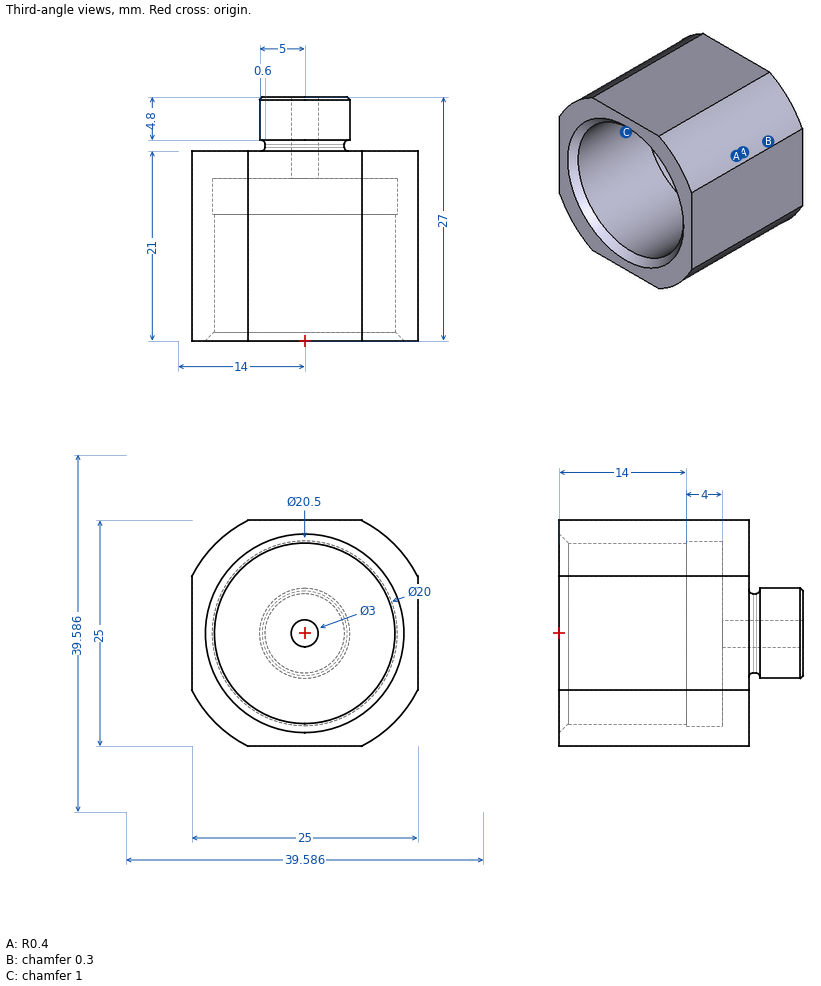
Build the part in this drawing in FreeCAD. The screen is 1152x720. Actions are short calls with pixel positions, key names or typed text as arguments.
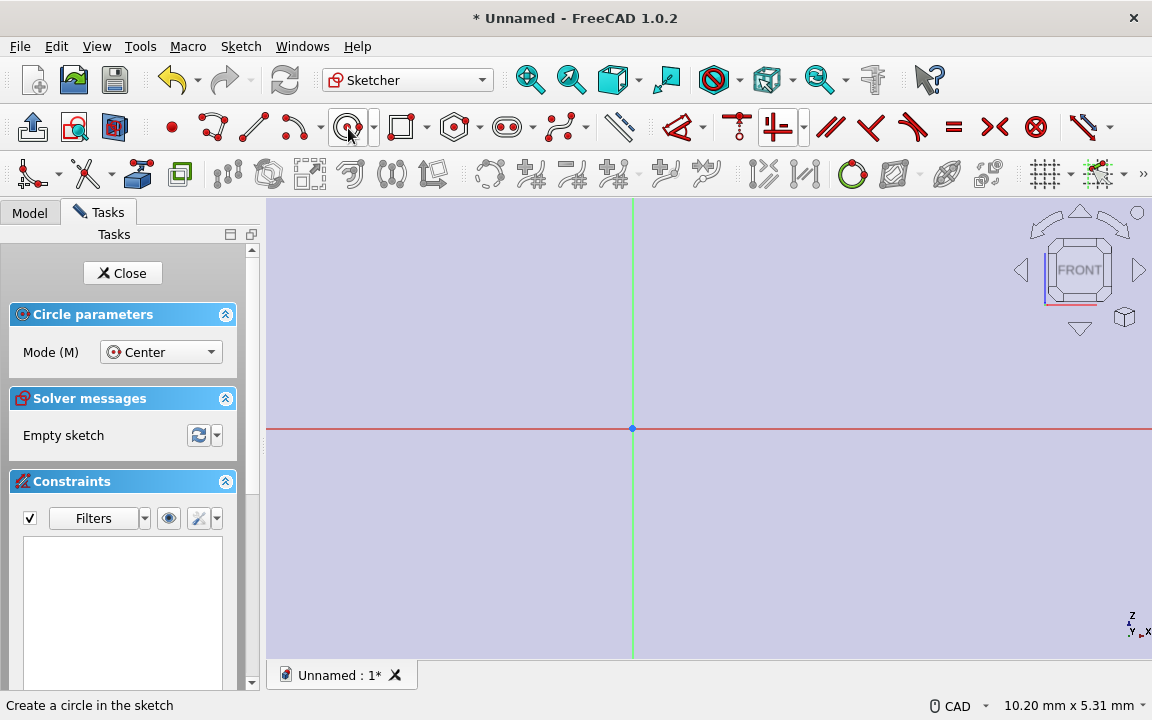
click(633, 428)
click(725, 336)
key(Escape)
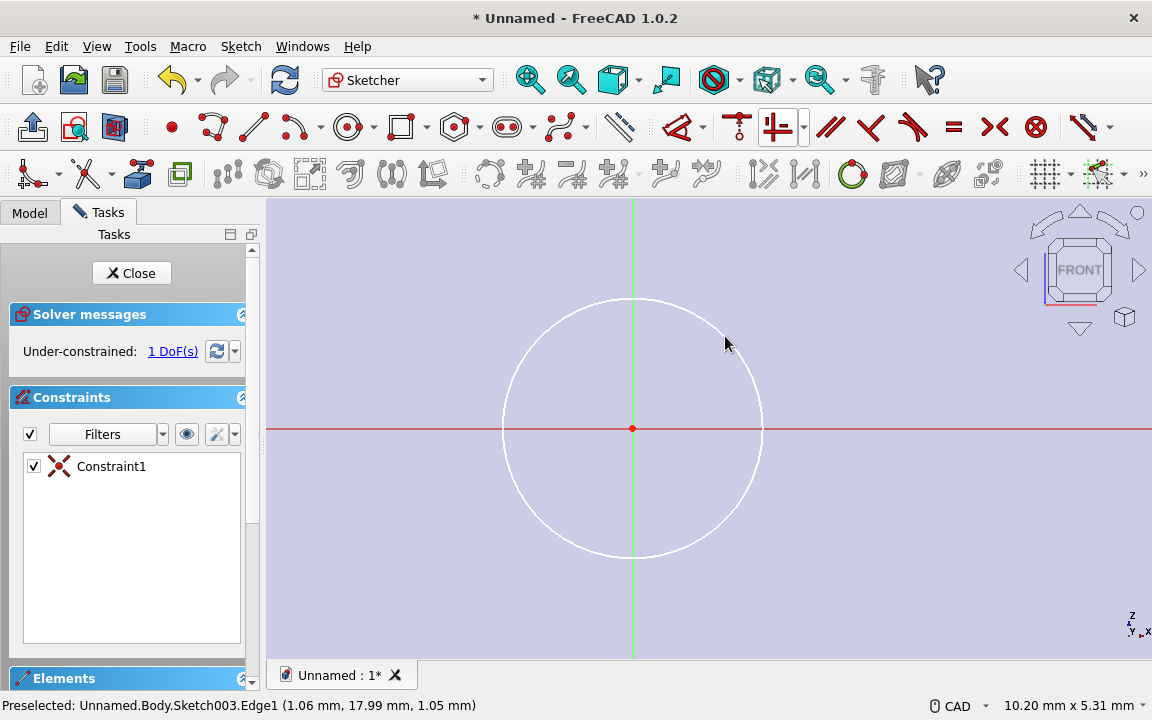
click(676, 128)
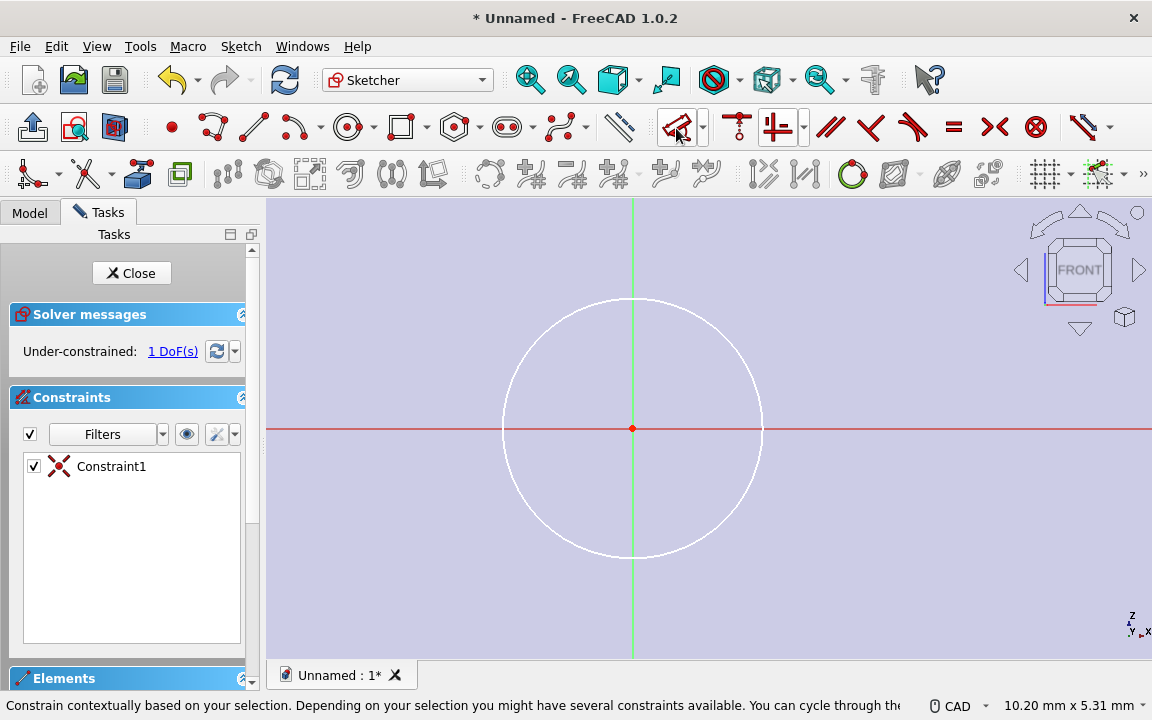
click(724, 336)
click(746, 313)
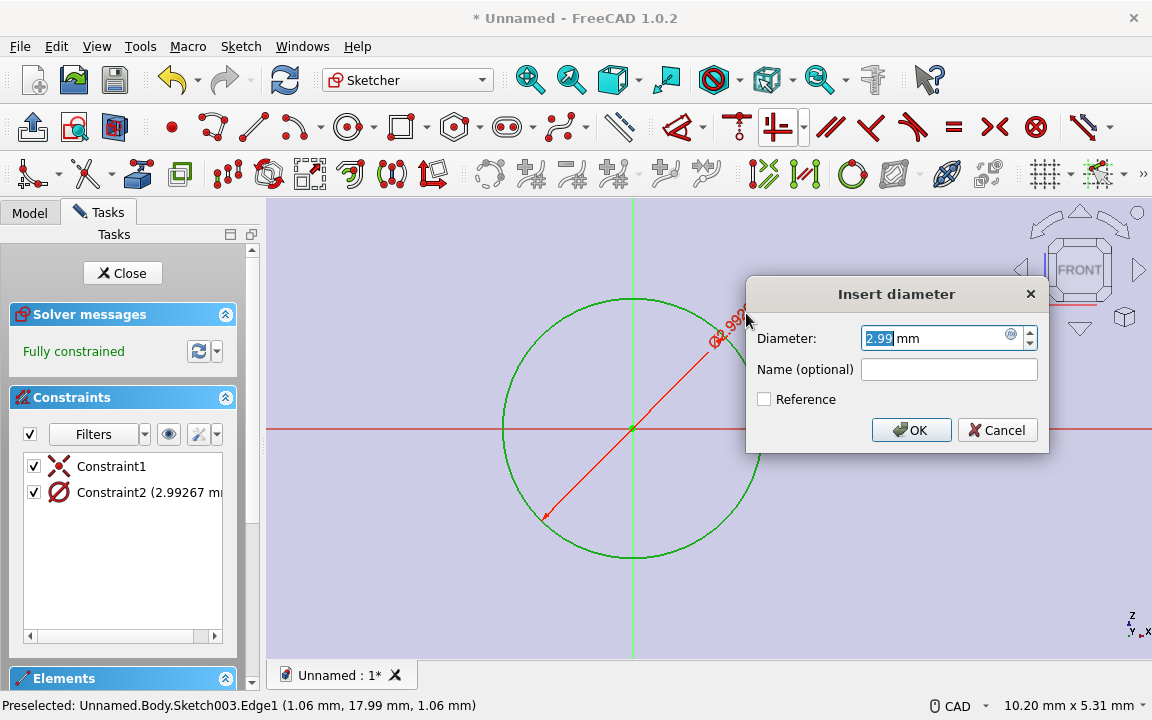
text(3)
key(Return)
key(Escape)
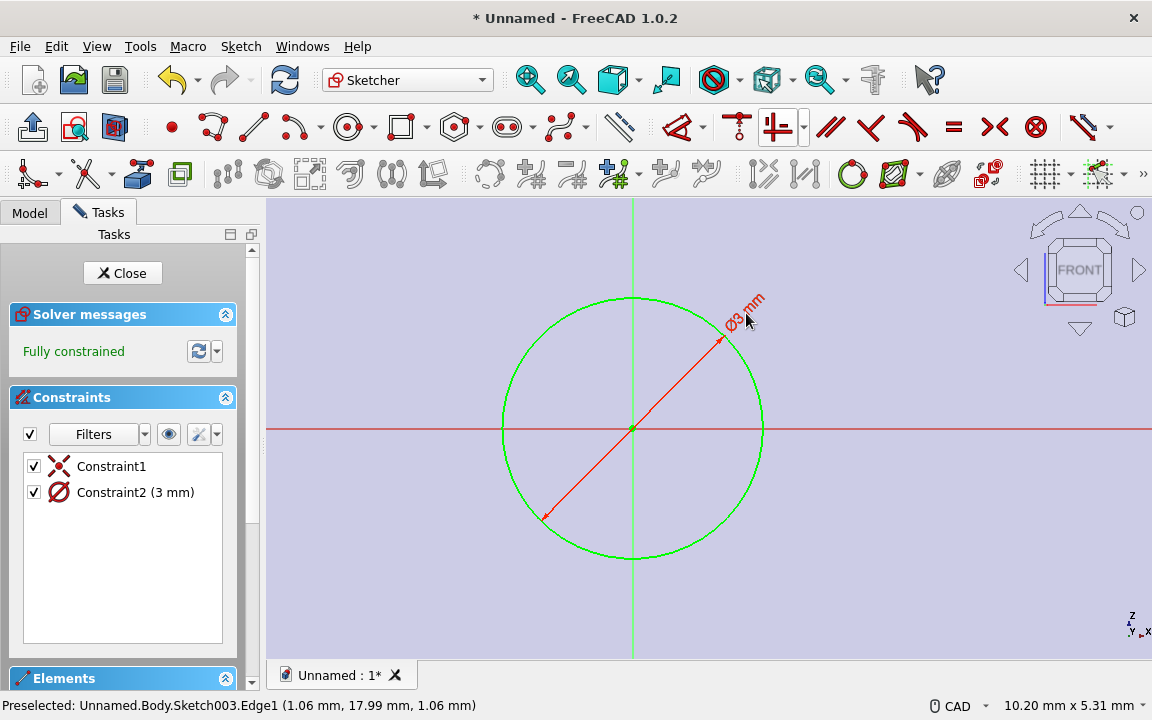
click(123, 273)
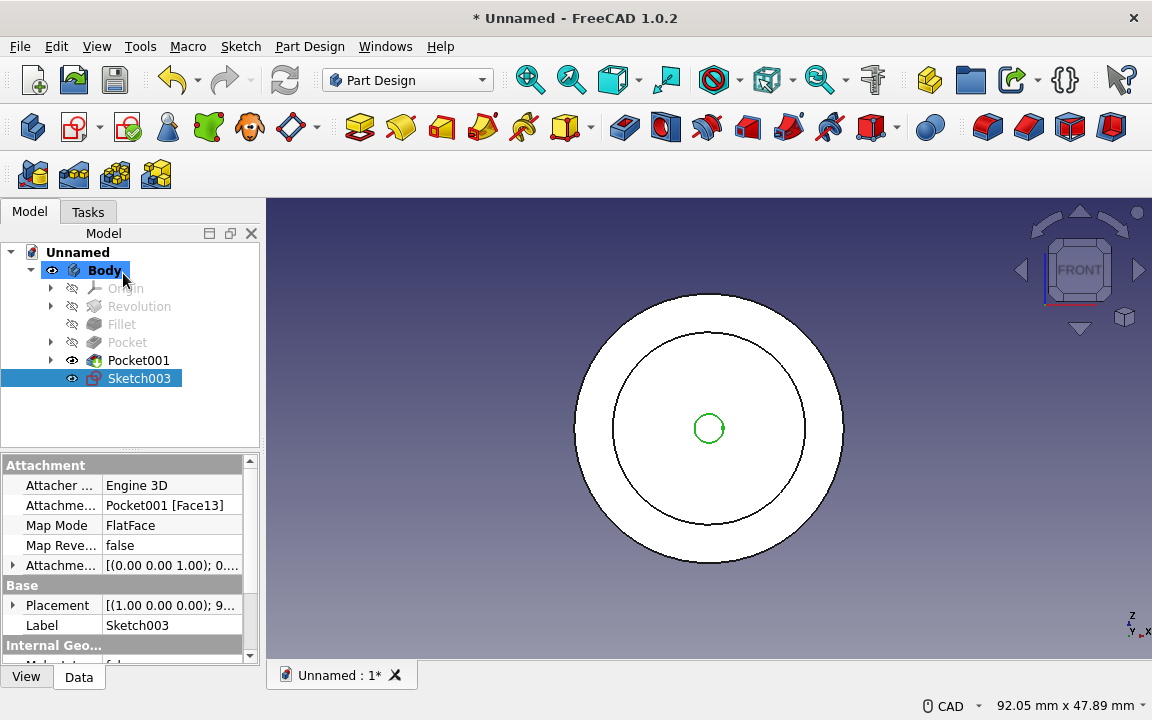
click(625, 128)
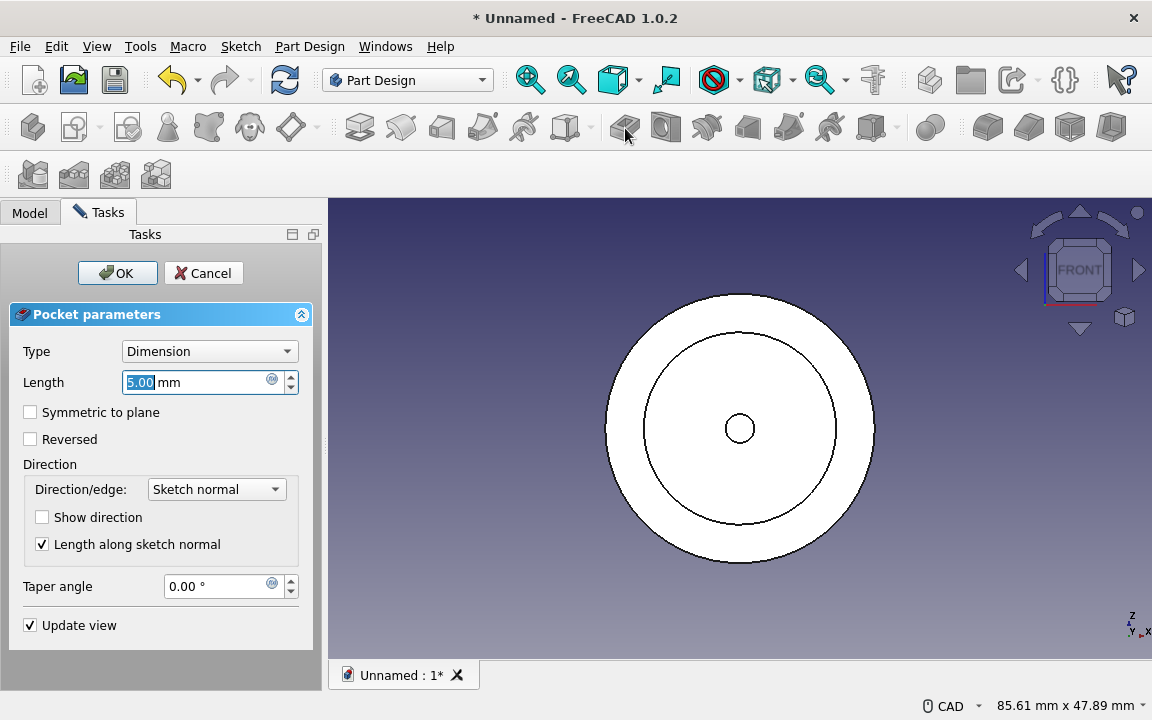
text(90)
key(Tab)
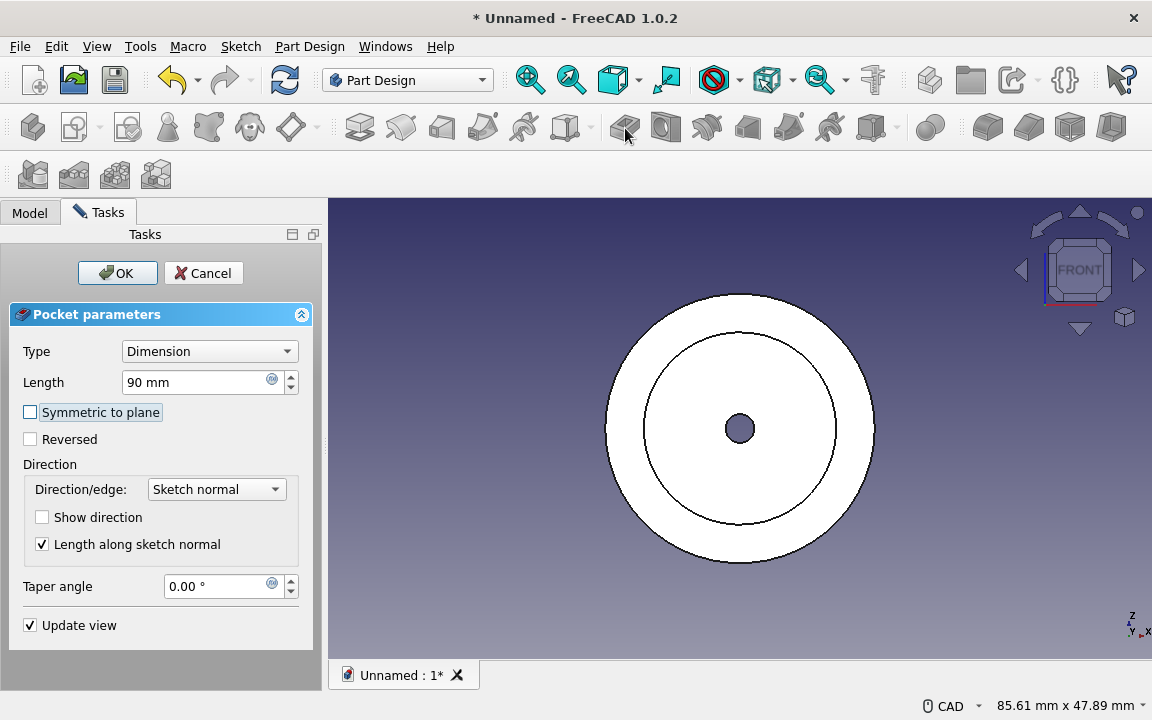
click(118, 273)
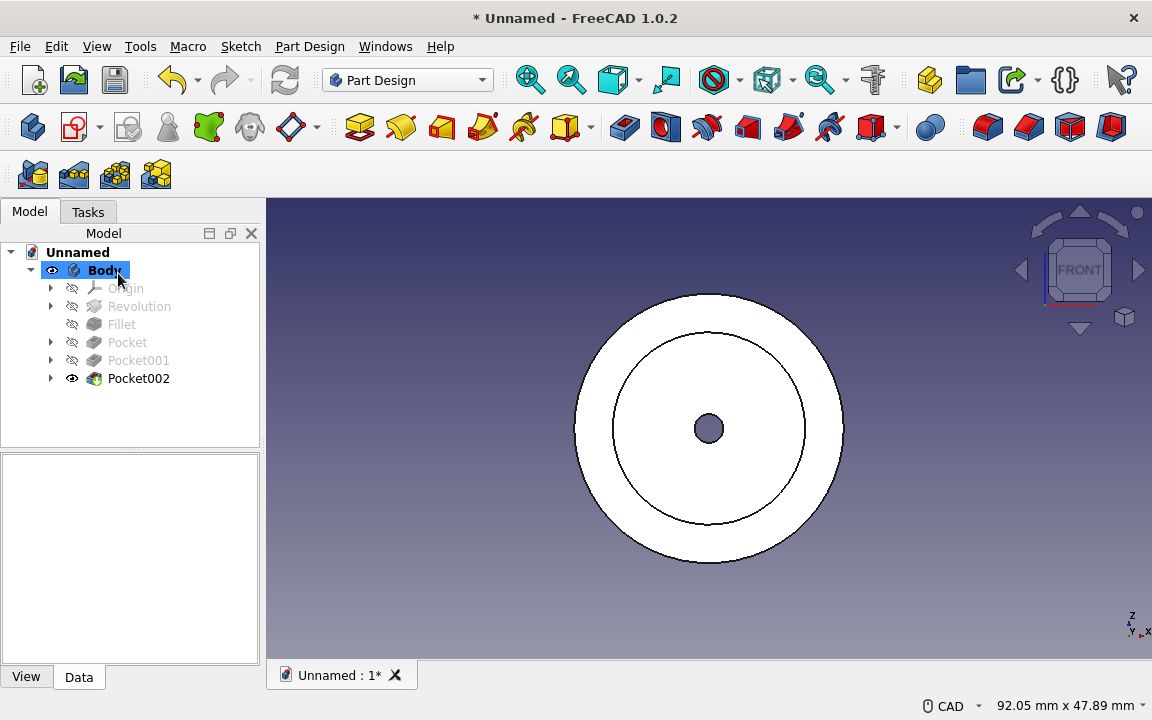
key(0)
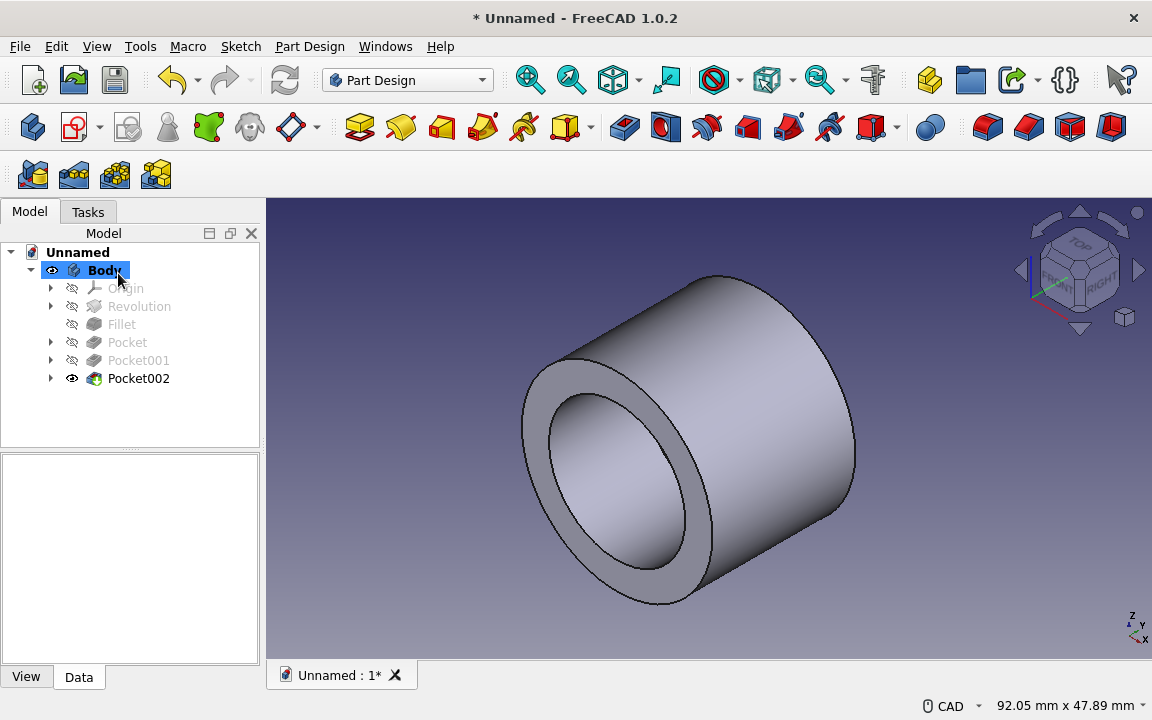
key(2)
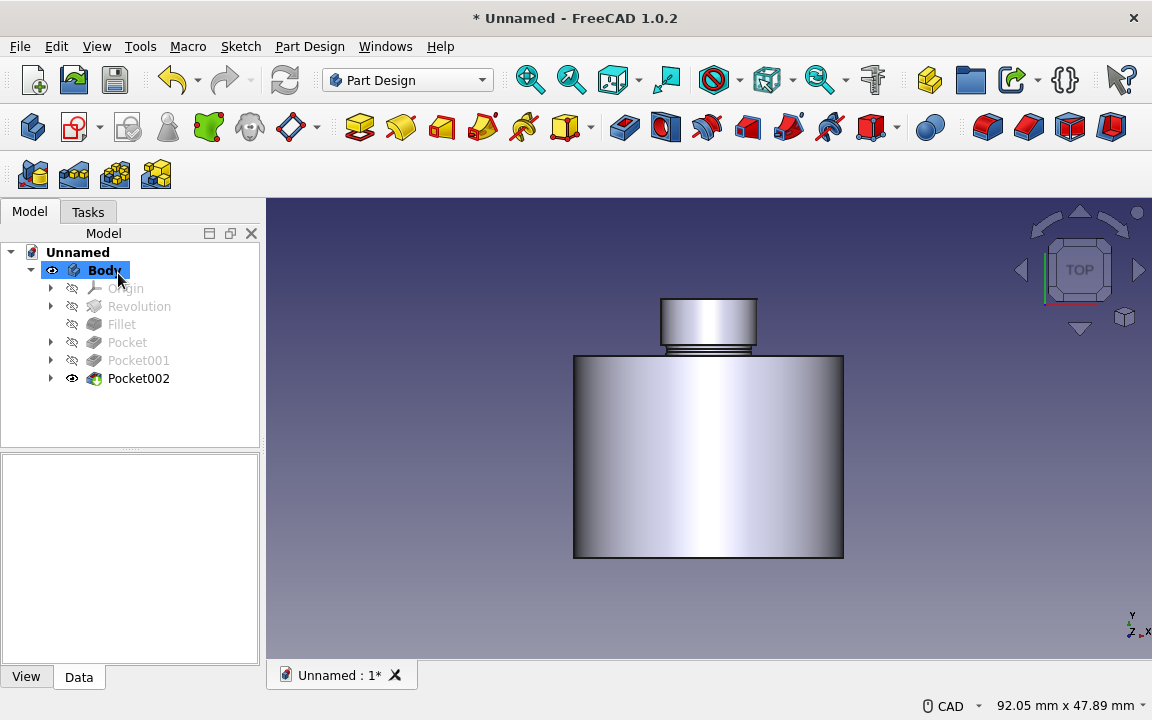
click(748, 298)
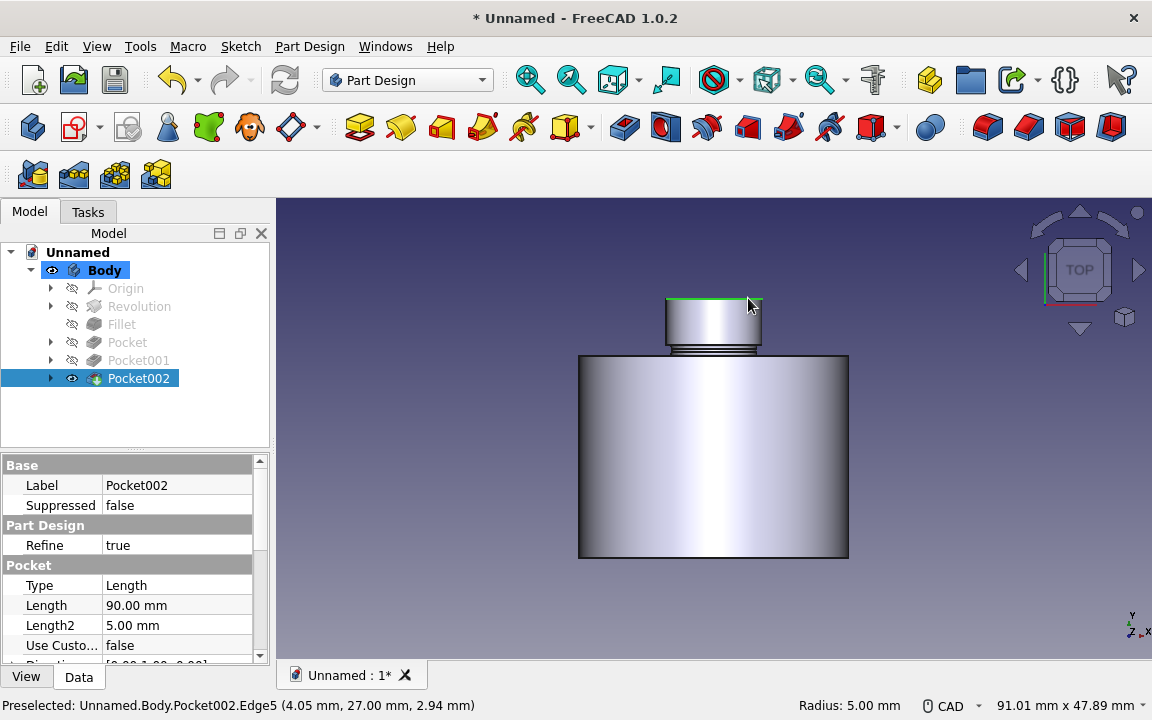
click(1029, 128)